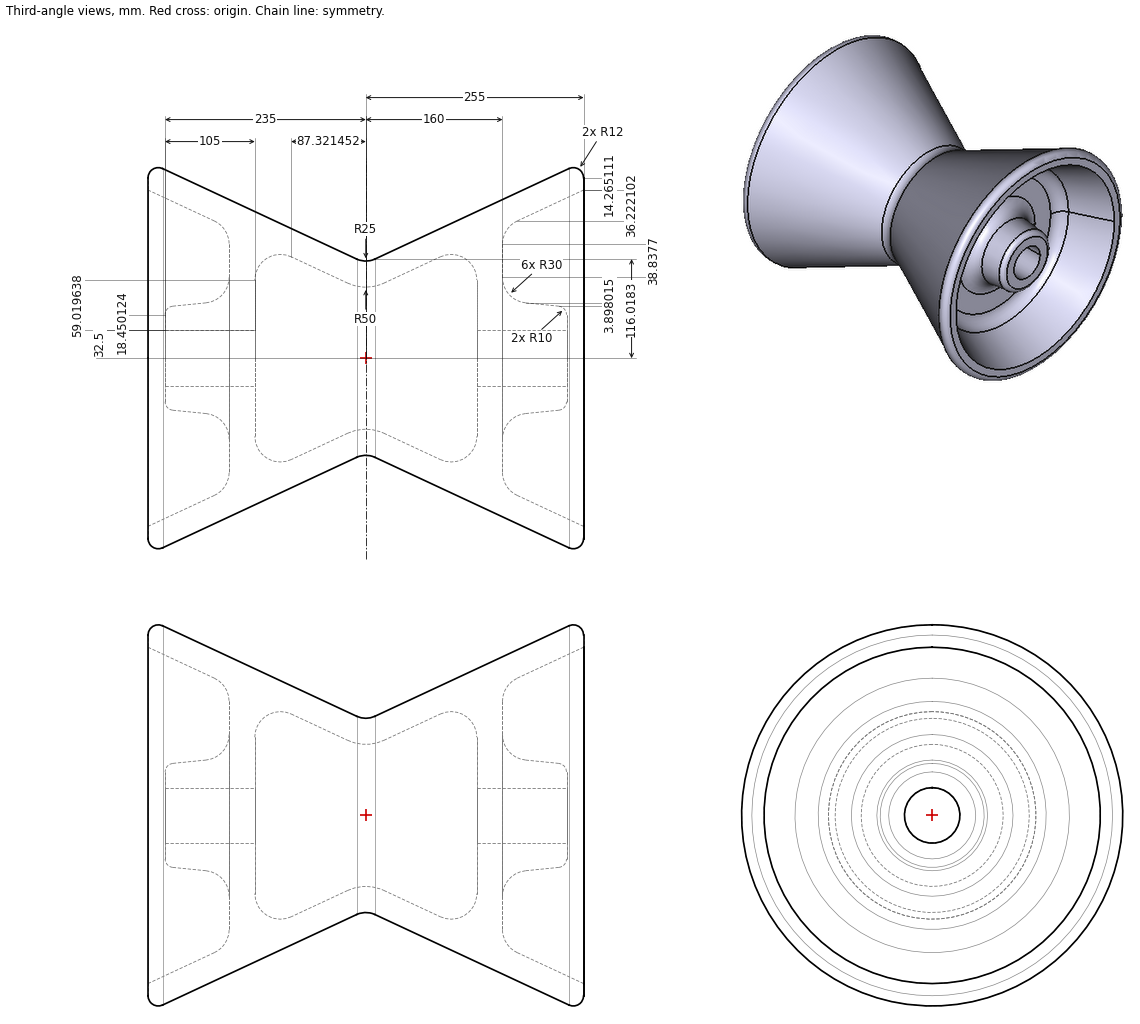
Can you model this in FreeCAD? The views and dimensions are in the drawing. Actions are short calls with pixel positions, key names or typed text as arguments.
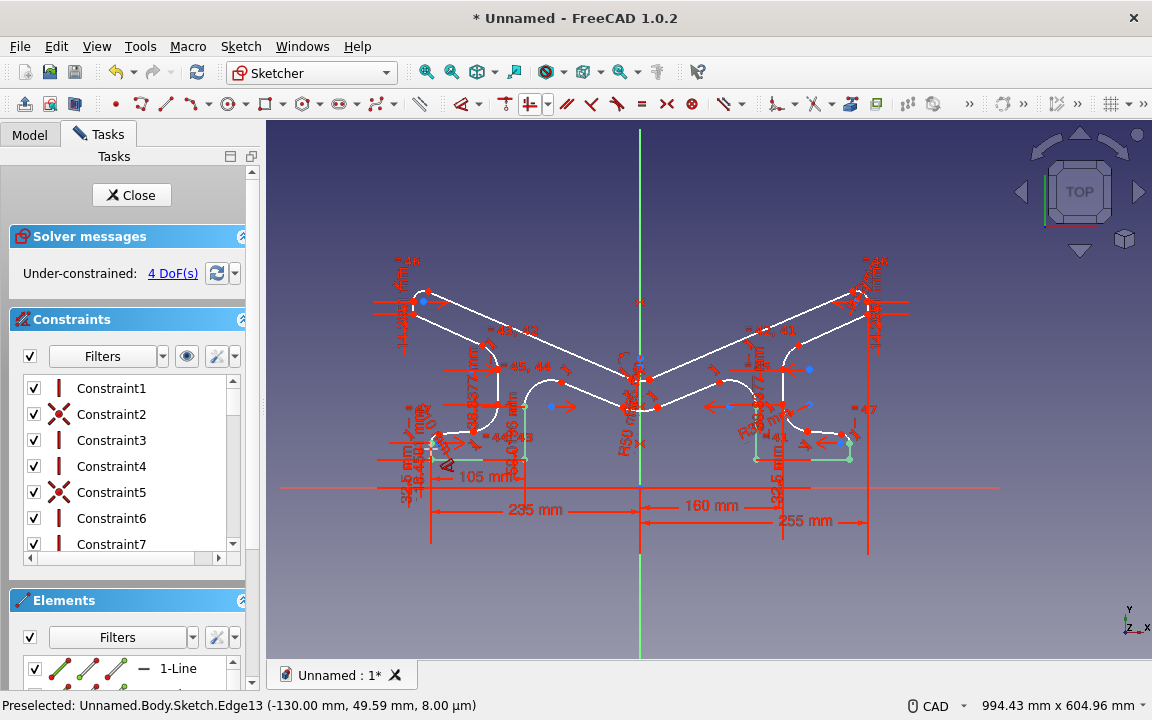
click(649, 379)
click(683, 459)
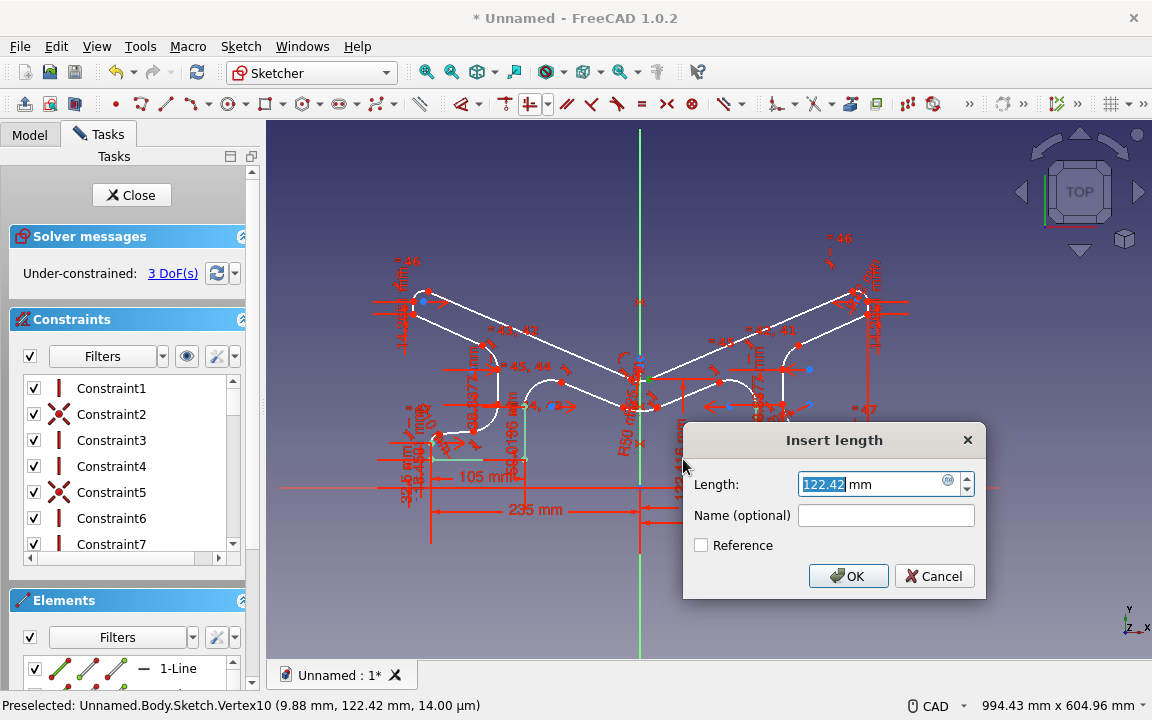
text(116.0183)
key(Return)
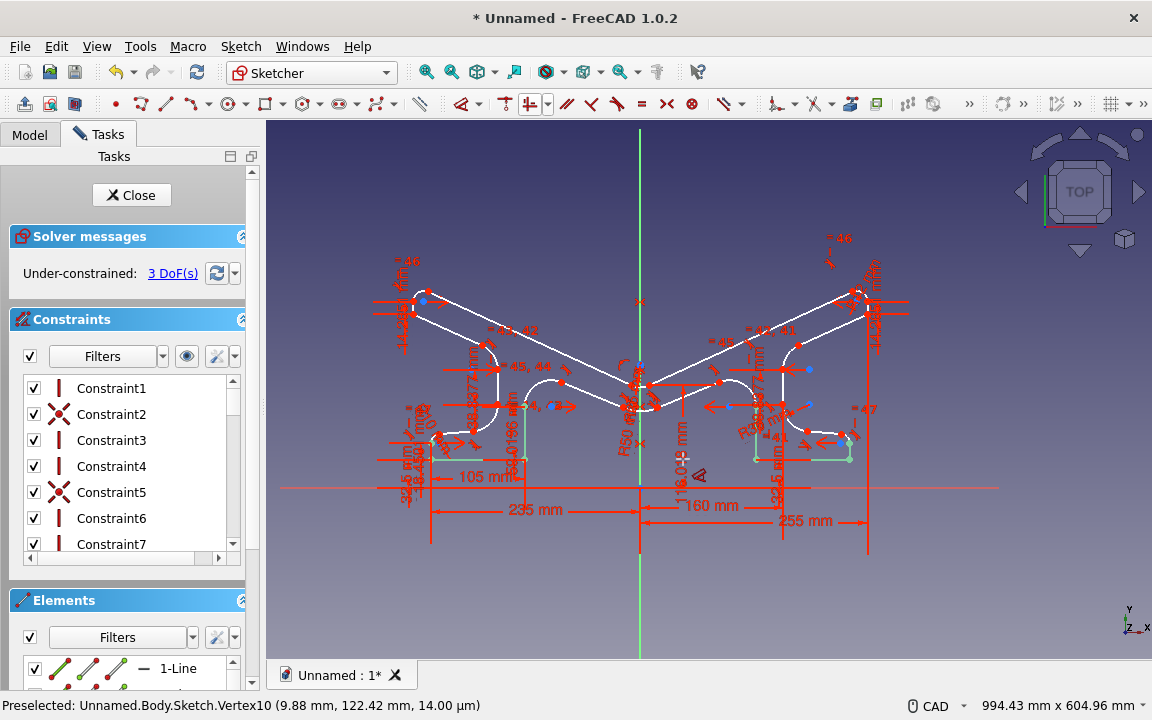
scroll(831, 433, up, 13)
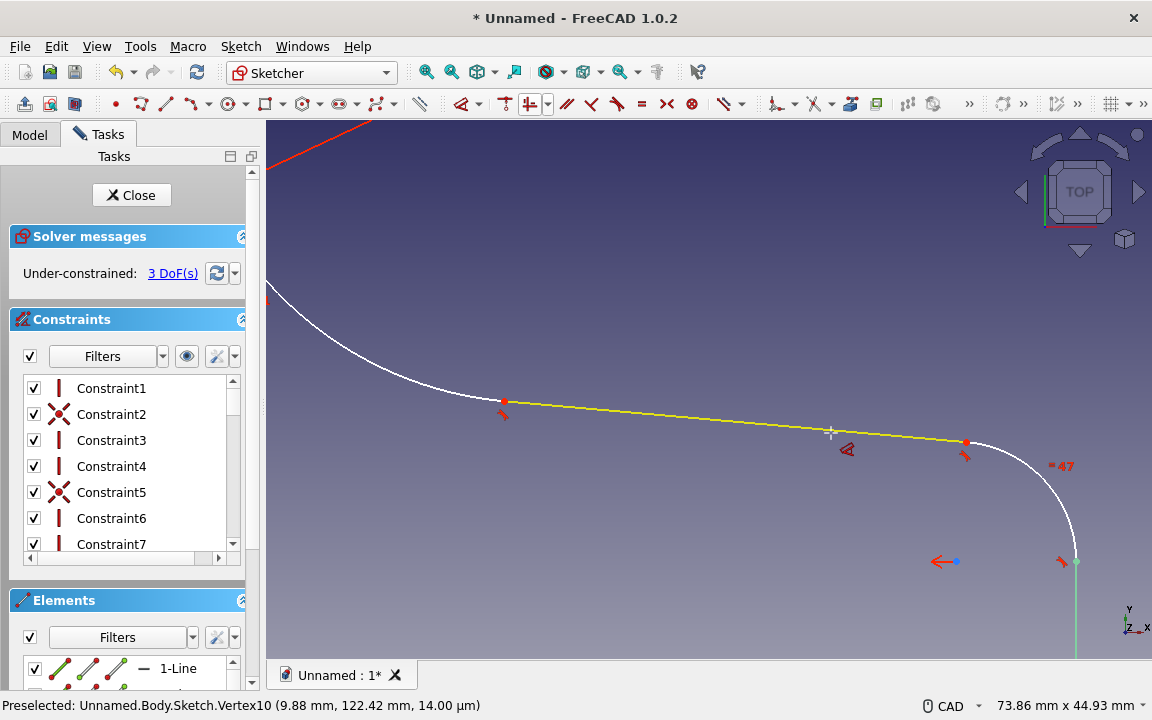
click(828, 430)
click(471, 422)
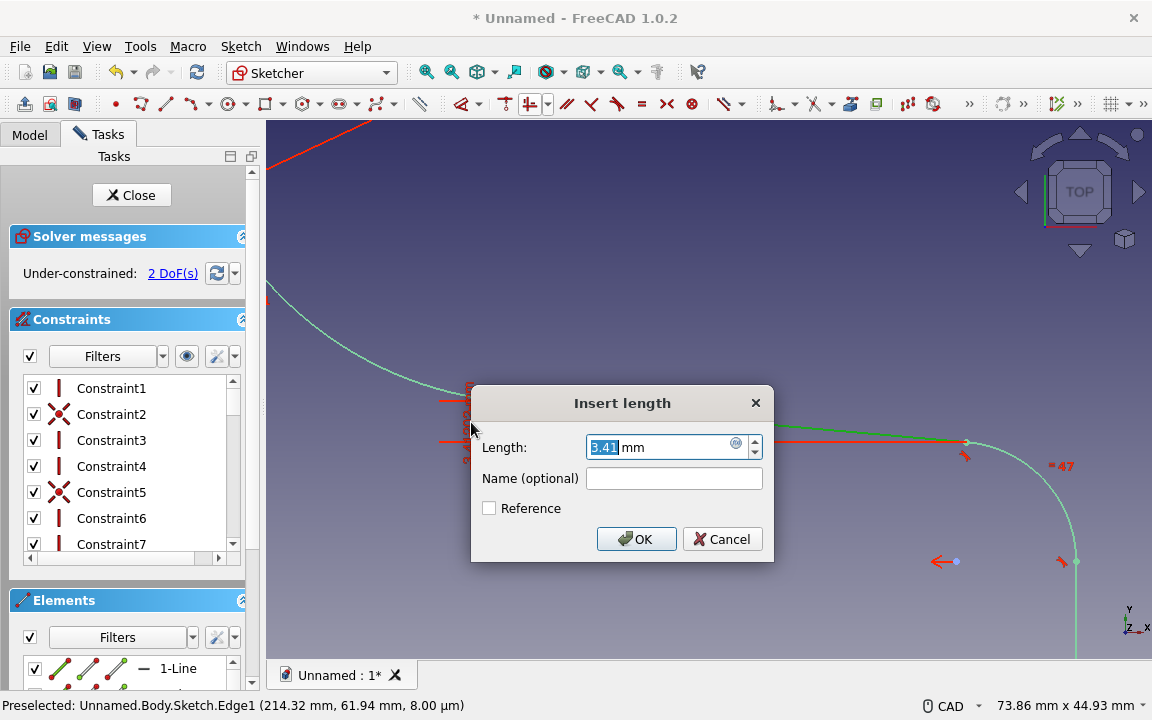
text(3.898015)
key(Return)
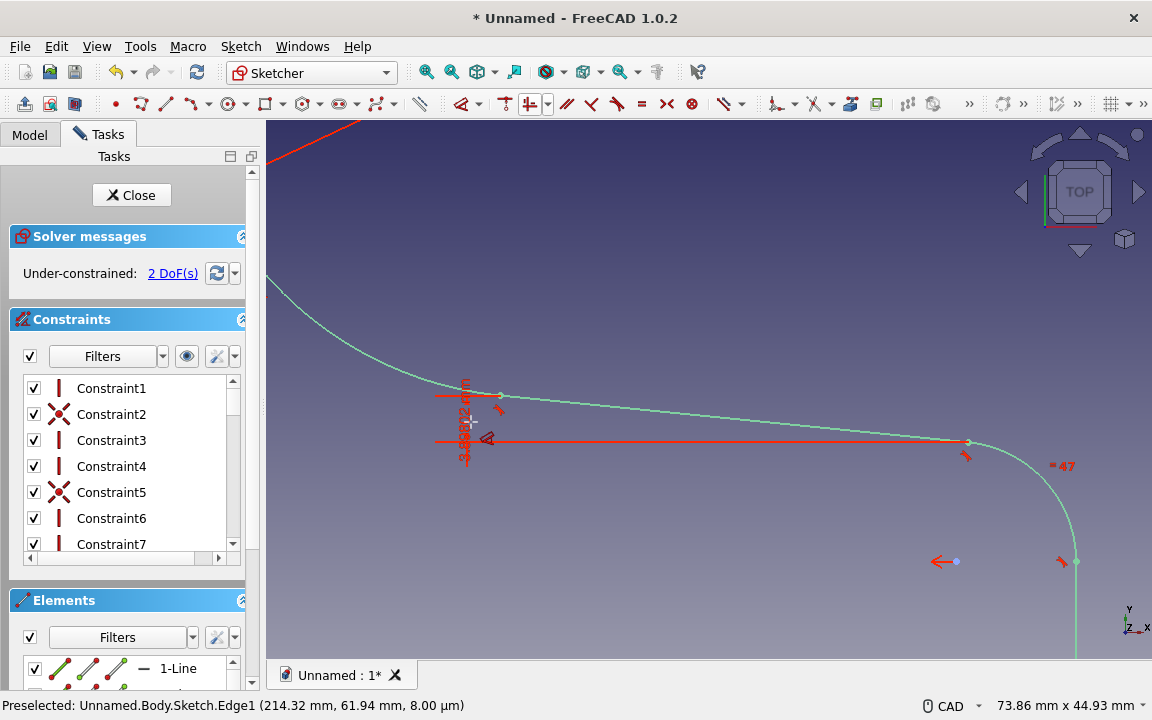
scroll(832, 433, down, 13)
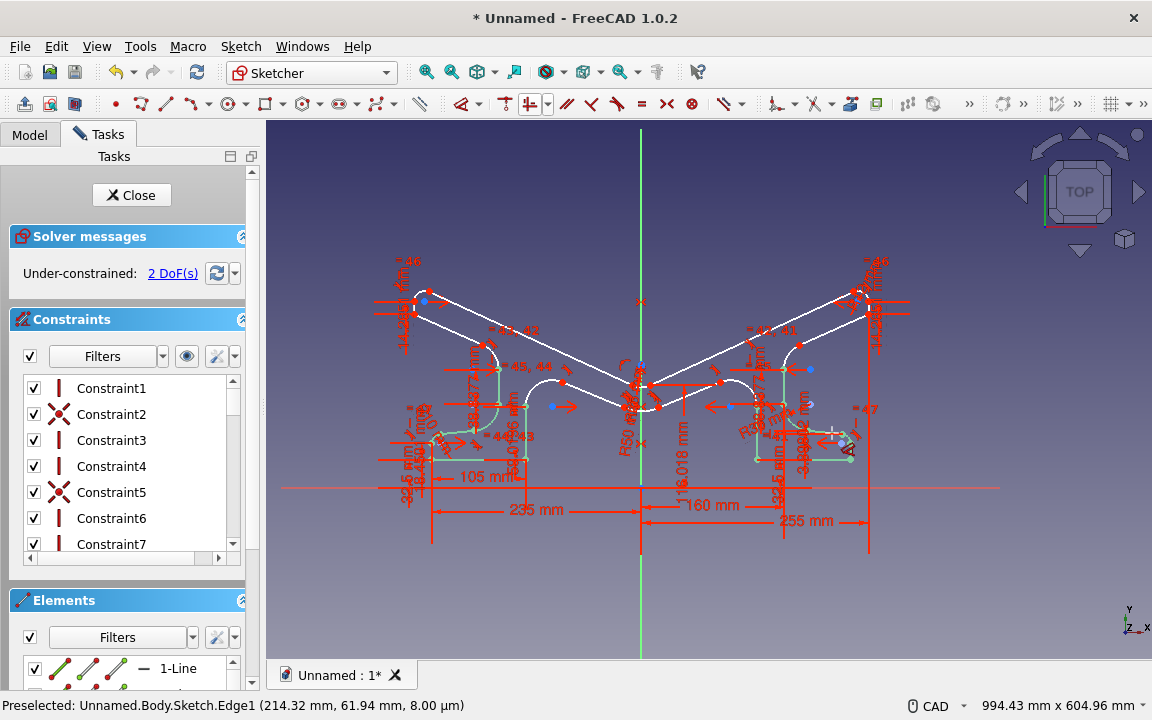
click(562, 382)
click(620, 522)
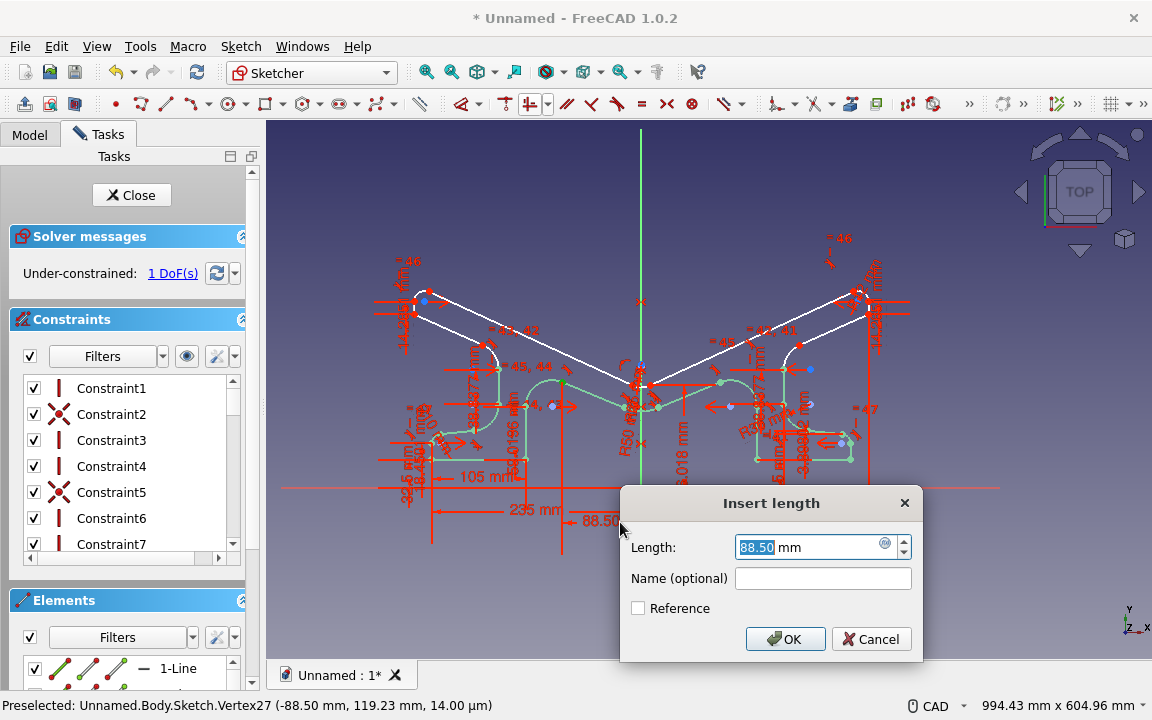
text(87.321452)
key(Return)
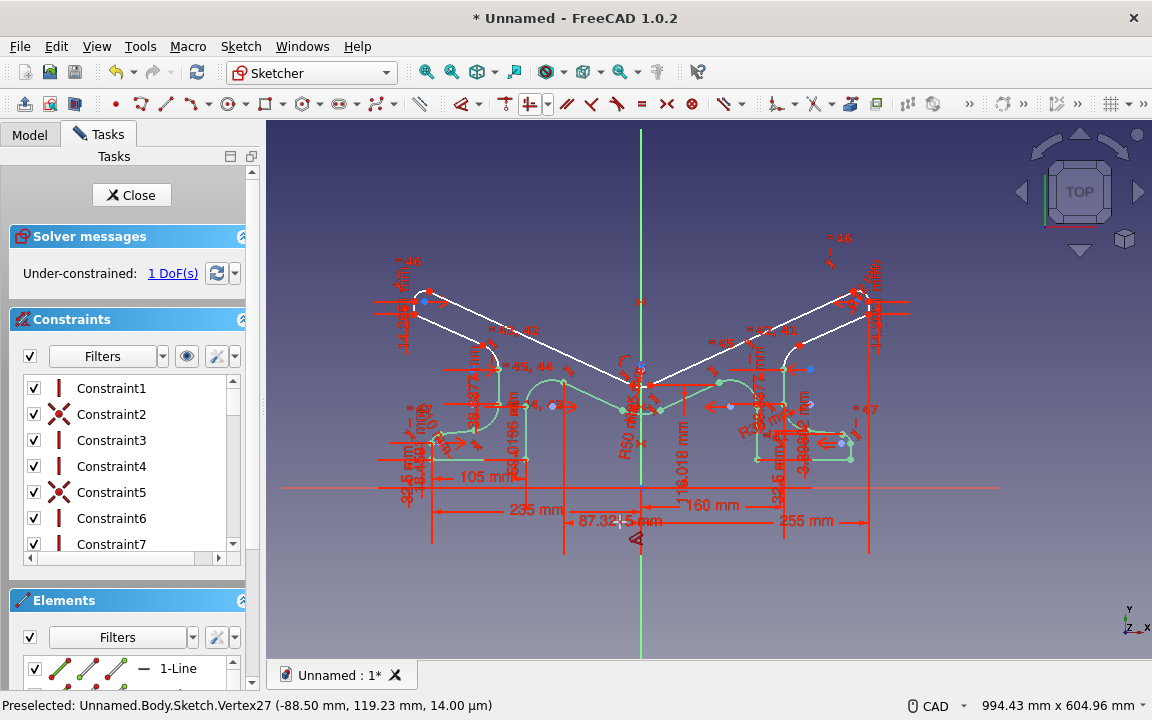
scroll(820, 336, up, 2)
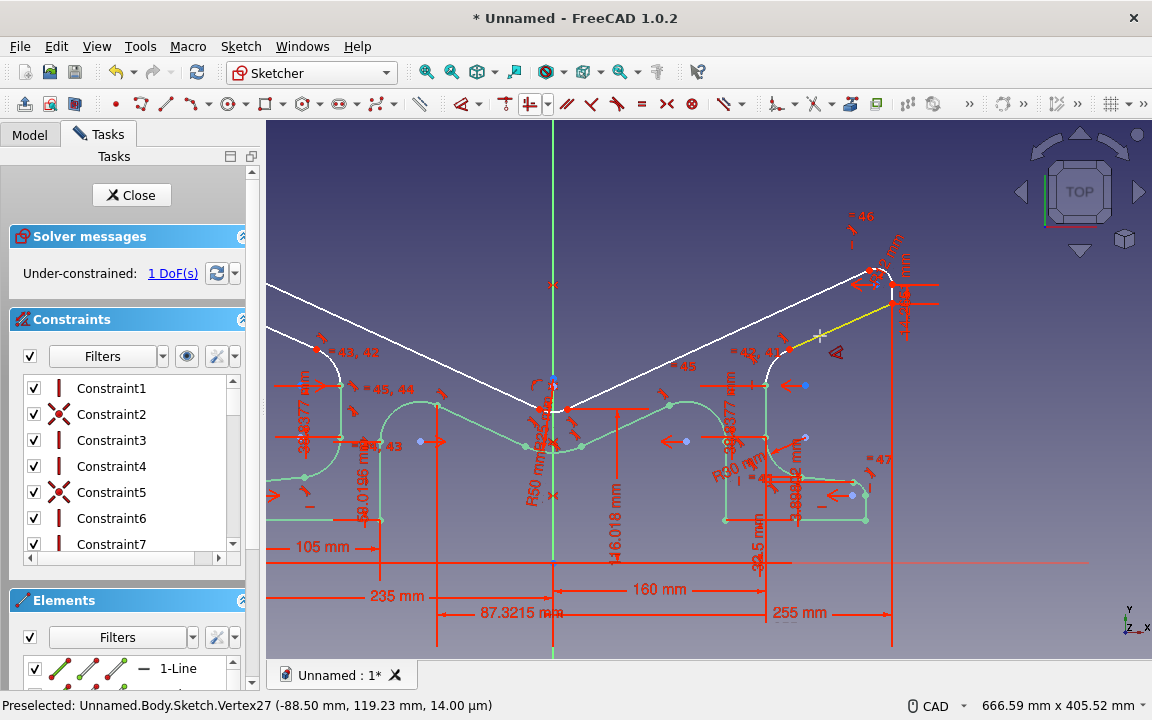
click(820, 336)
click(926, 327)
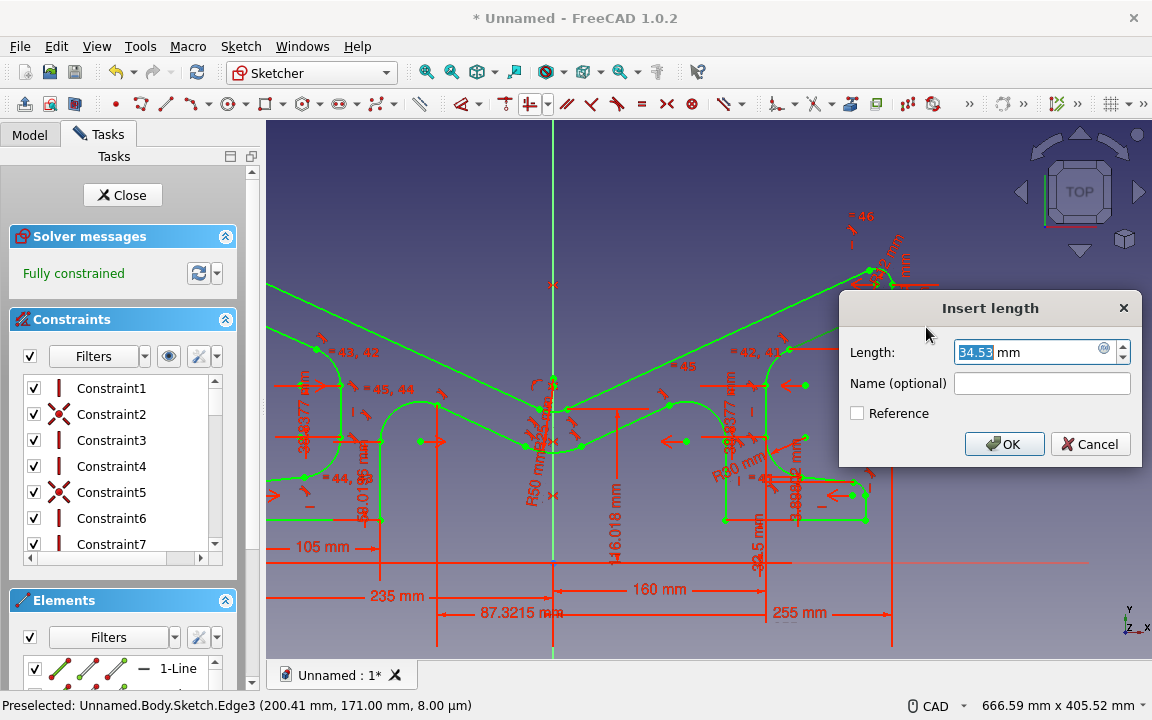
text(36.222102)
key(Return)
key(Escape)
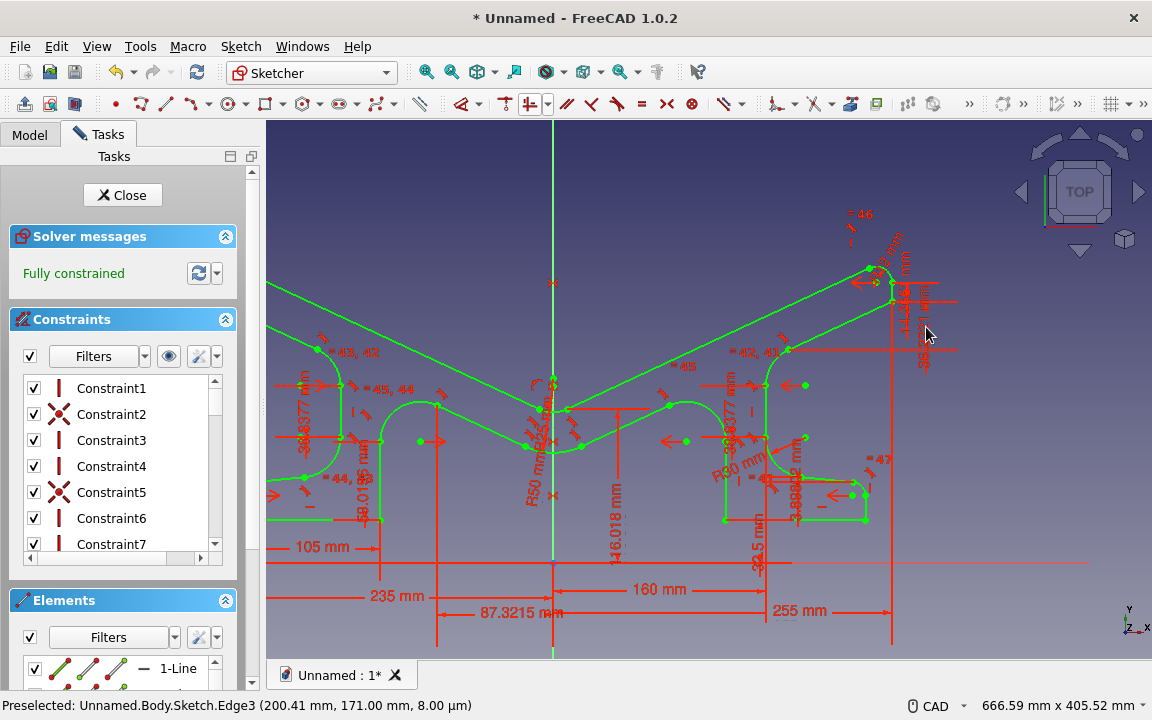
click(123, 195)